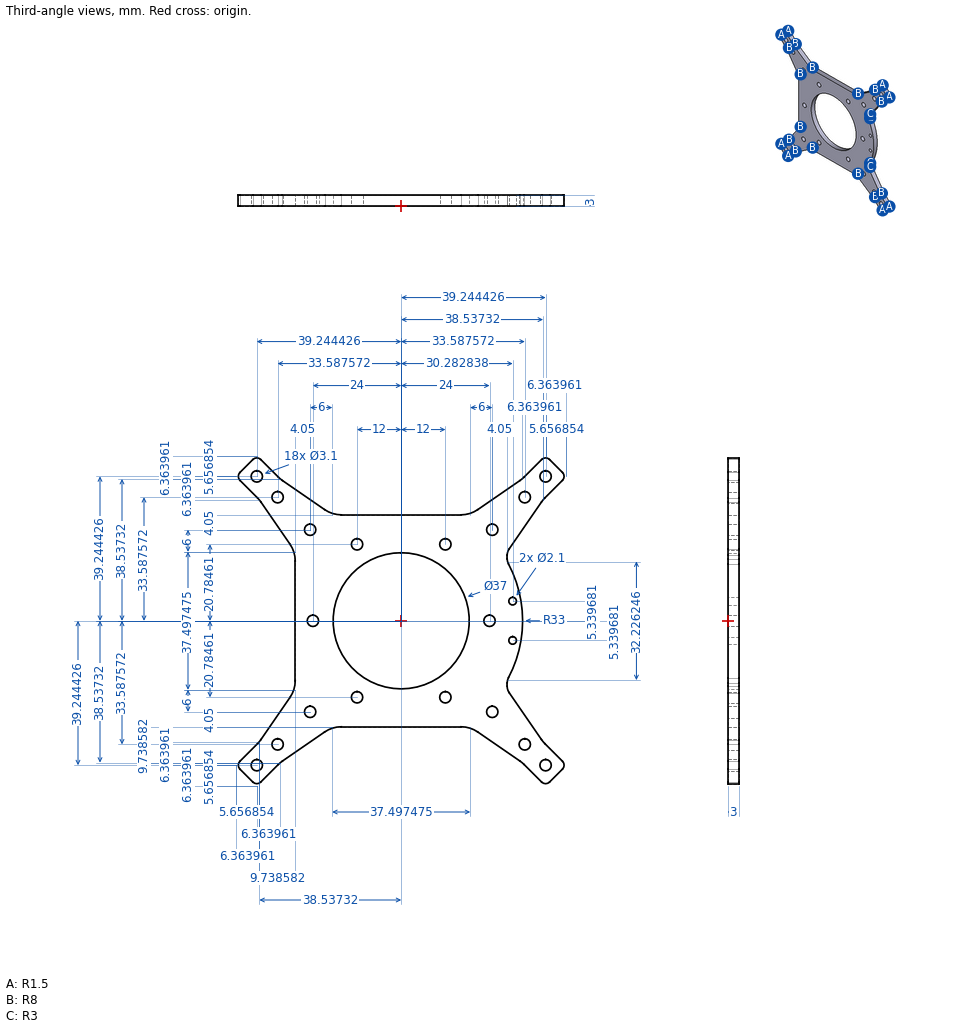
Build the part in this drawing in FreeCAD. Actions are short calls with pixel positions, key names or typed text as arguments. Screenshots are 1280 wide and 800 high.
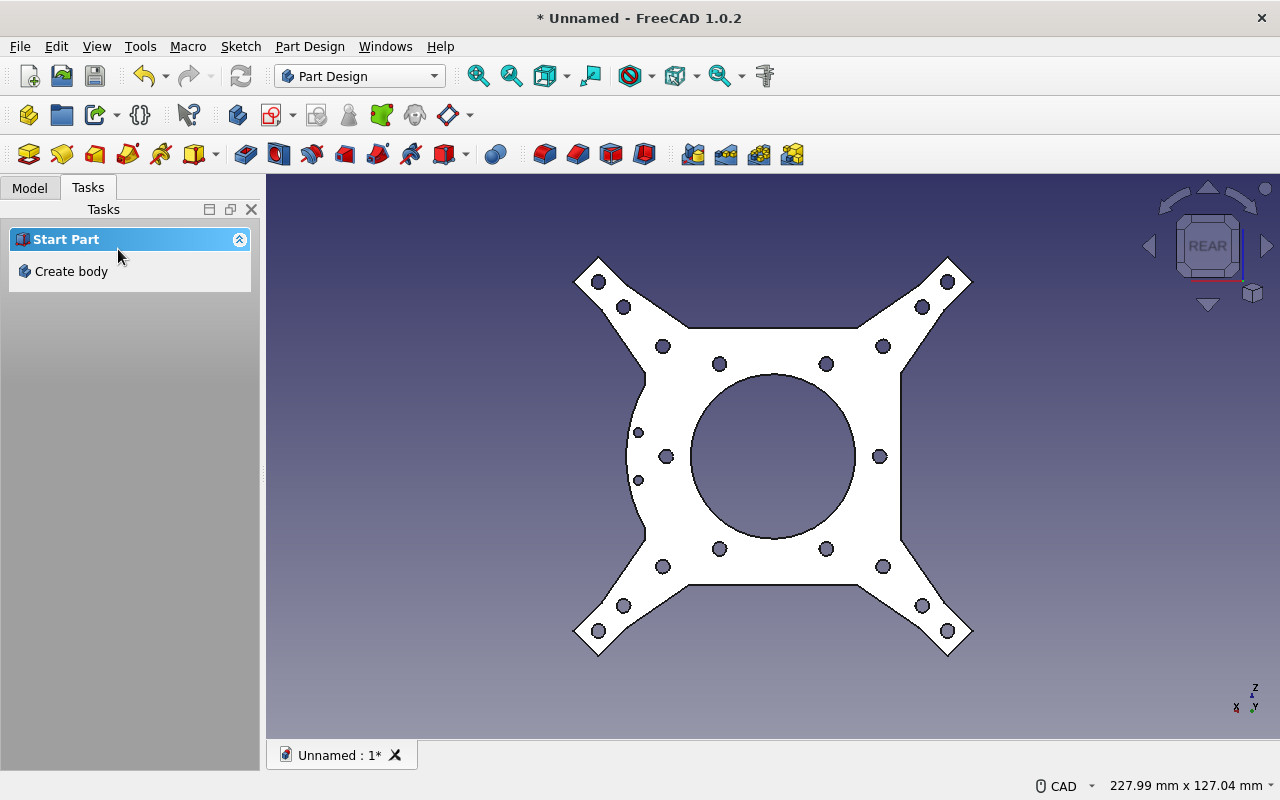
scroll(598, 655, up, 6)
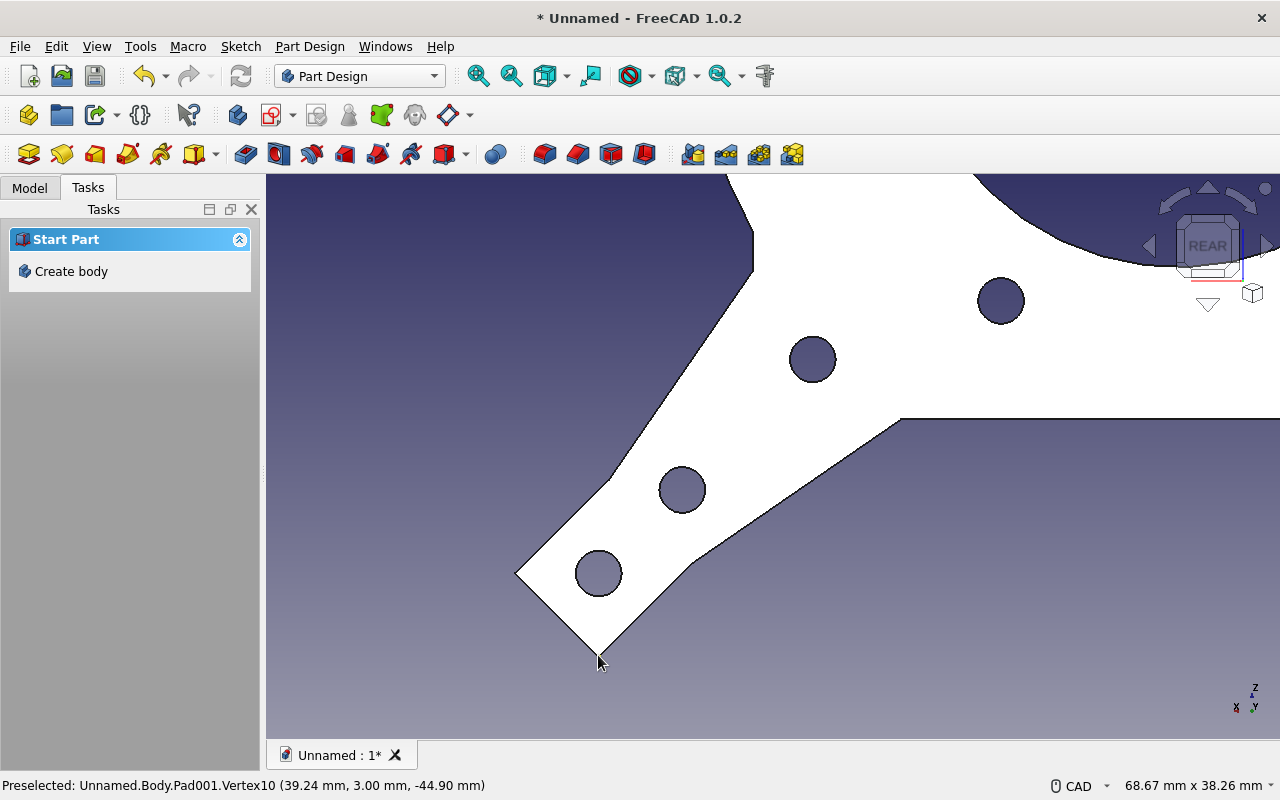
click(479, 76)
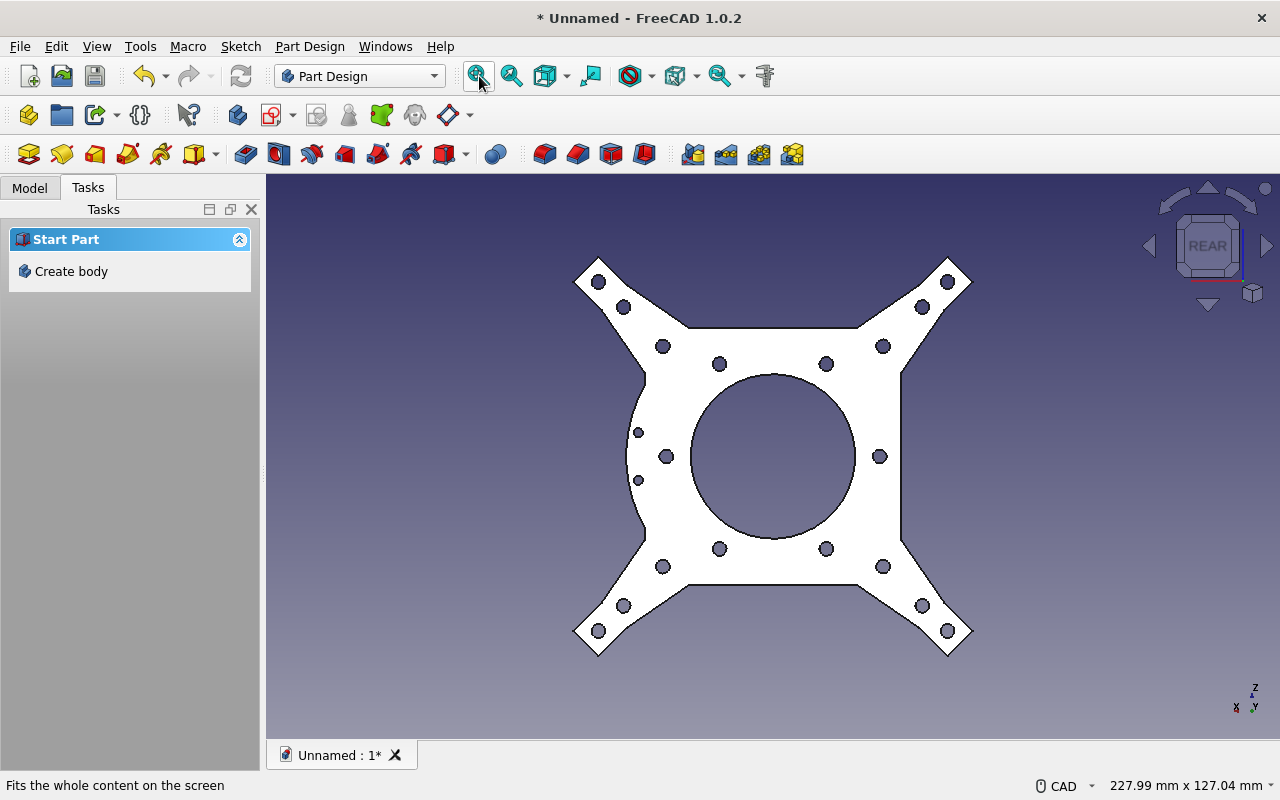
key(0)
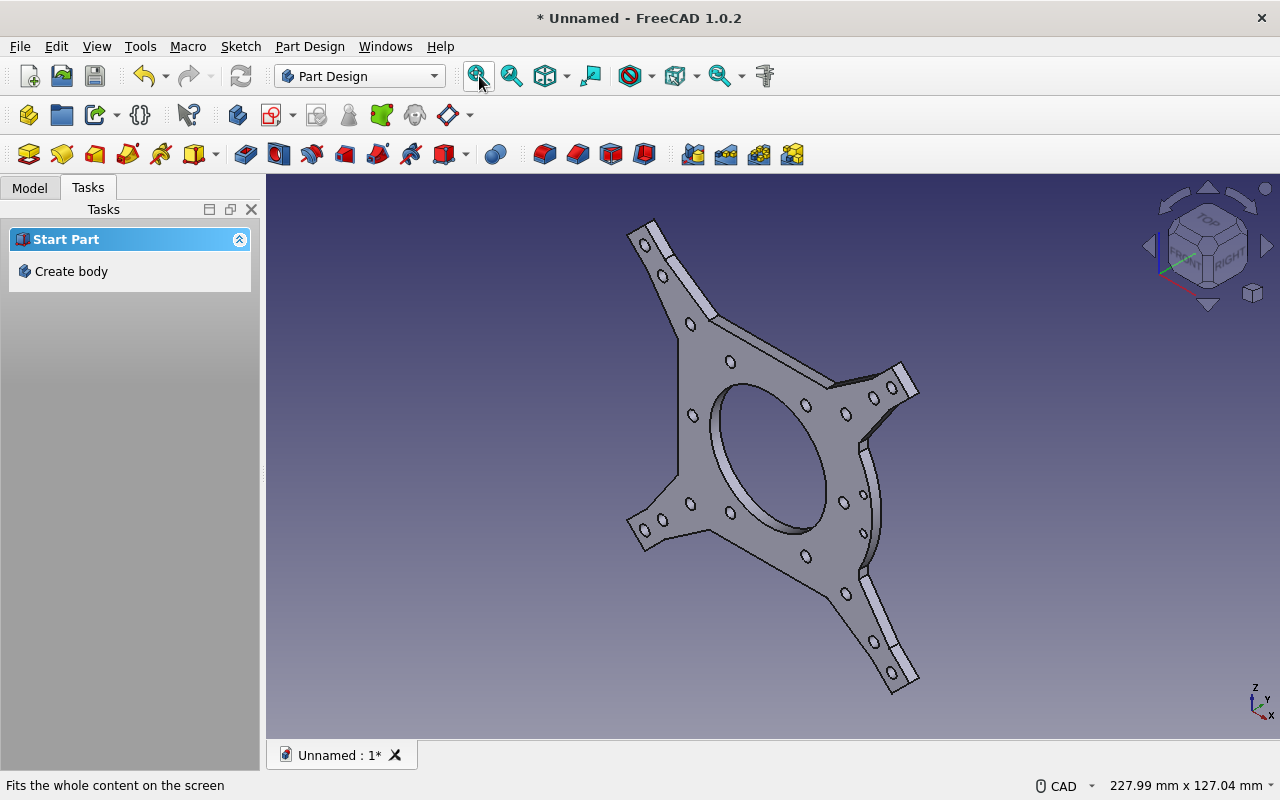
click(915, 679)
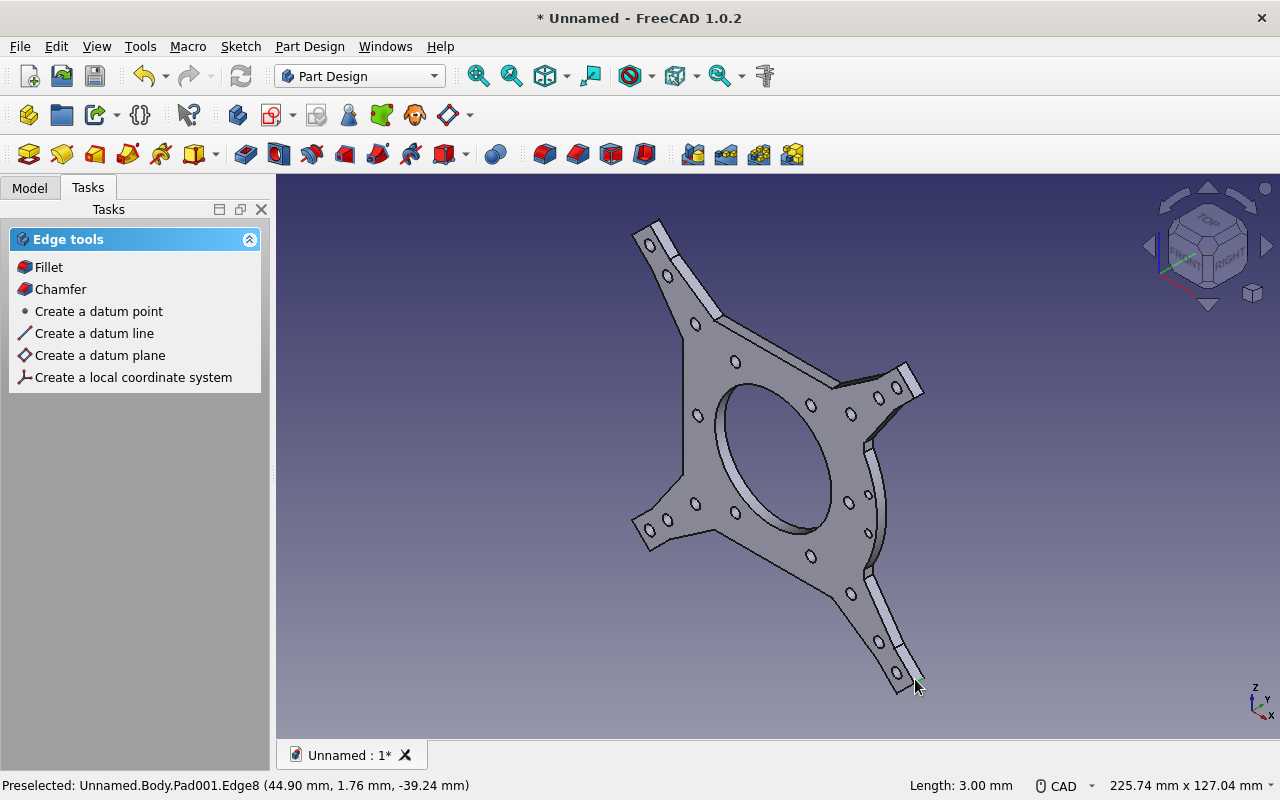
click(920, 394, ctrl)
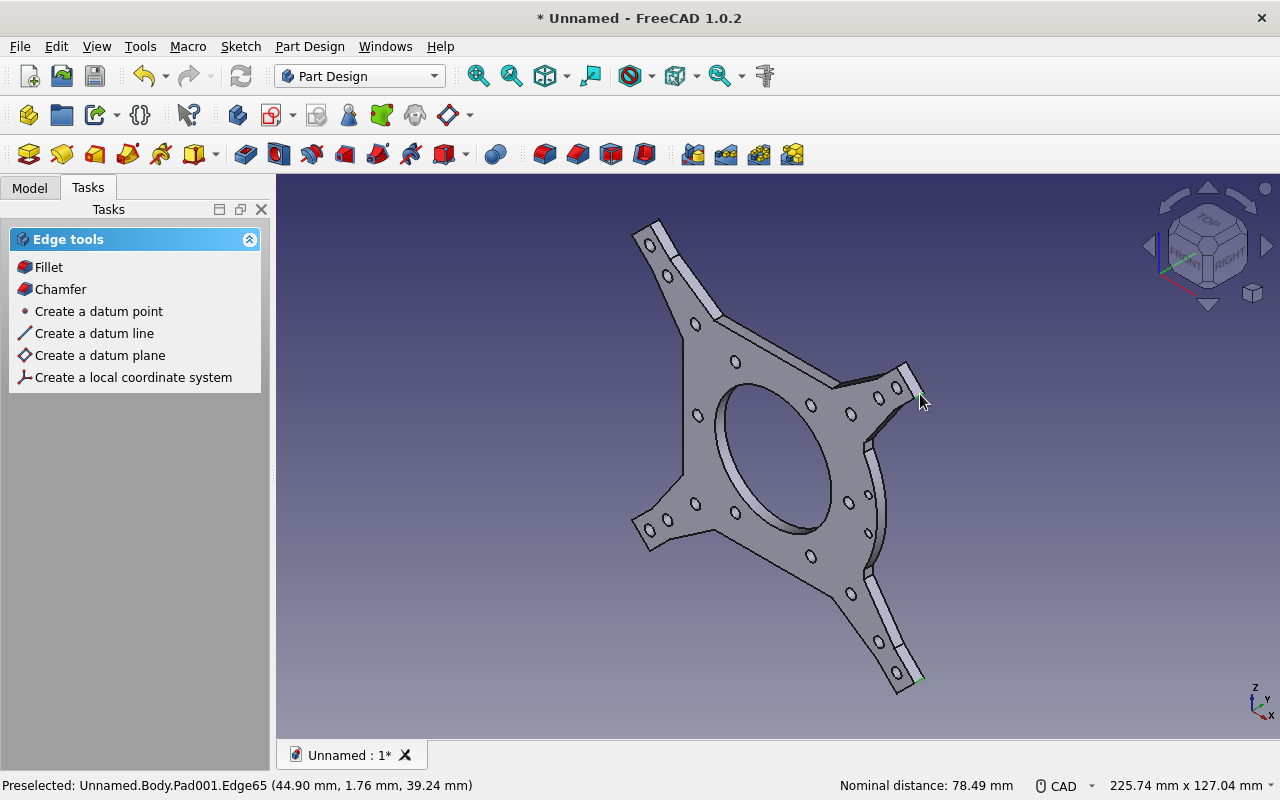
scroll(901, 690, up, 6)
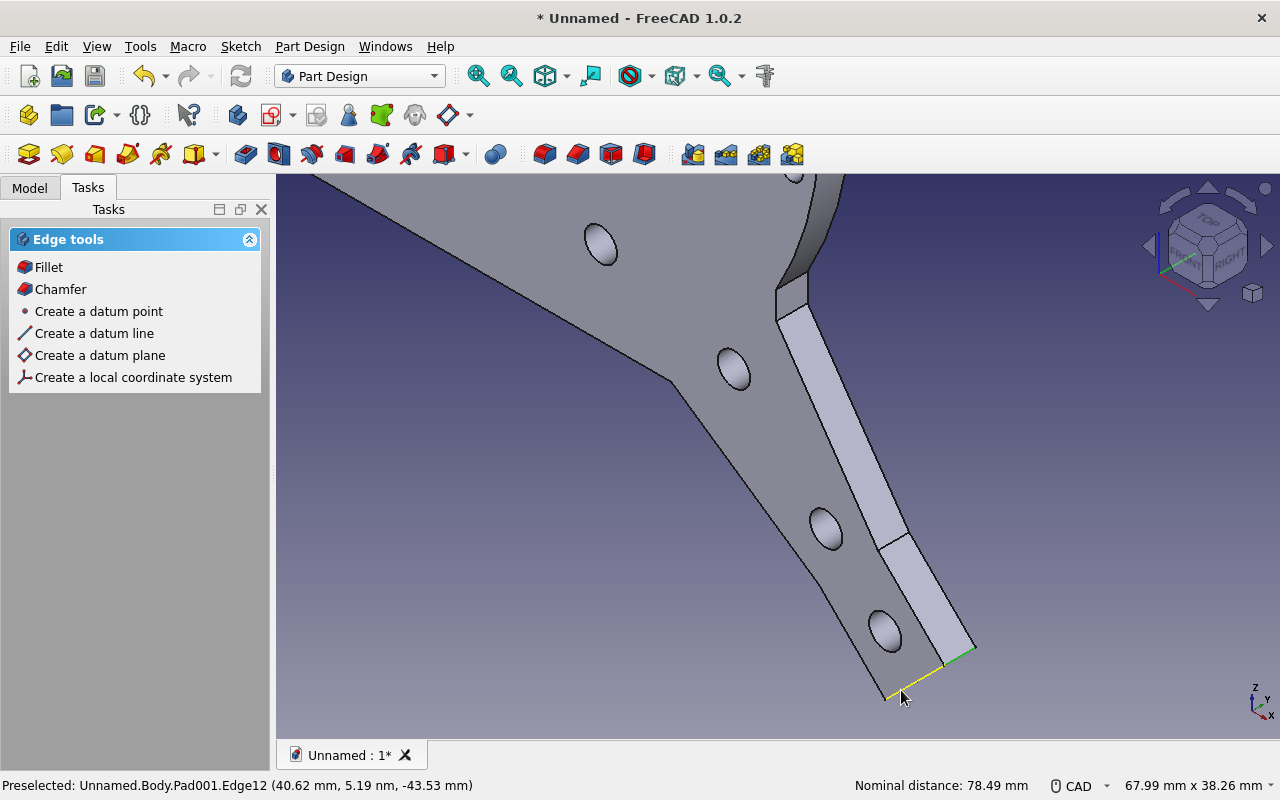
click(479, 76)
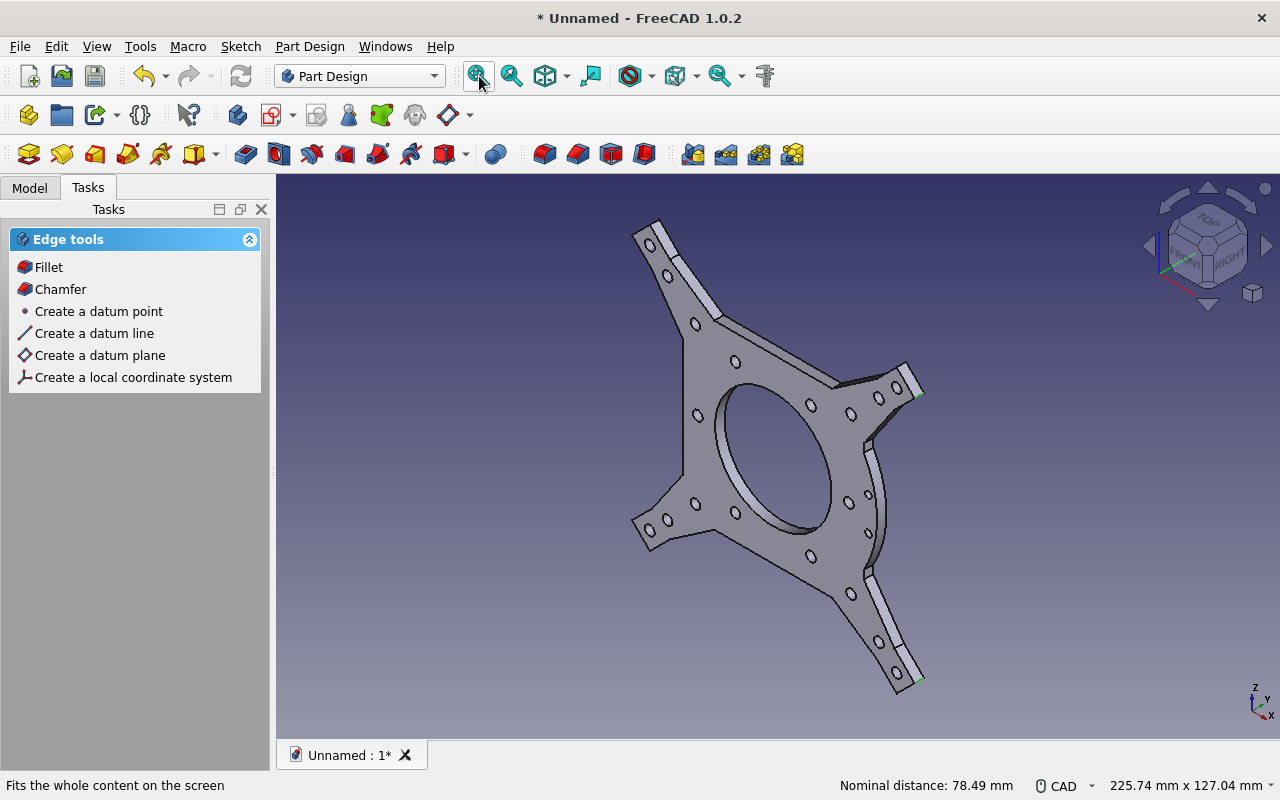
key(2)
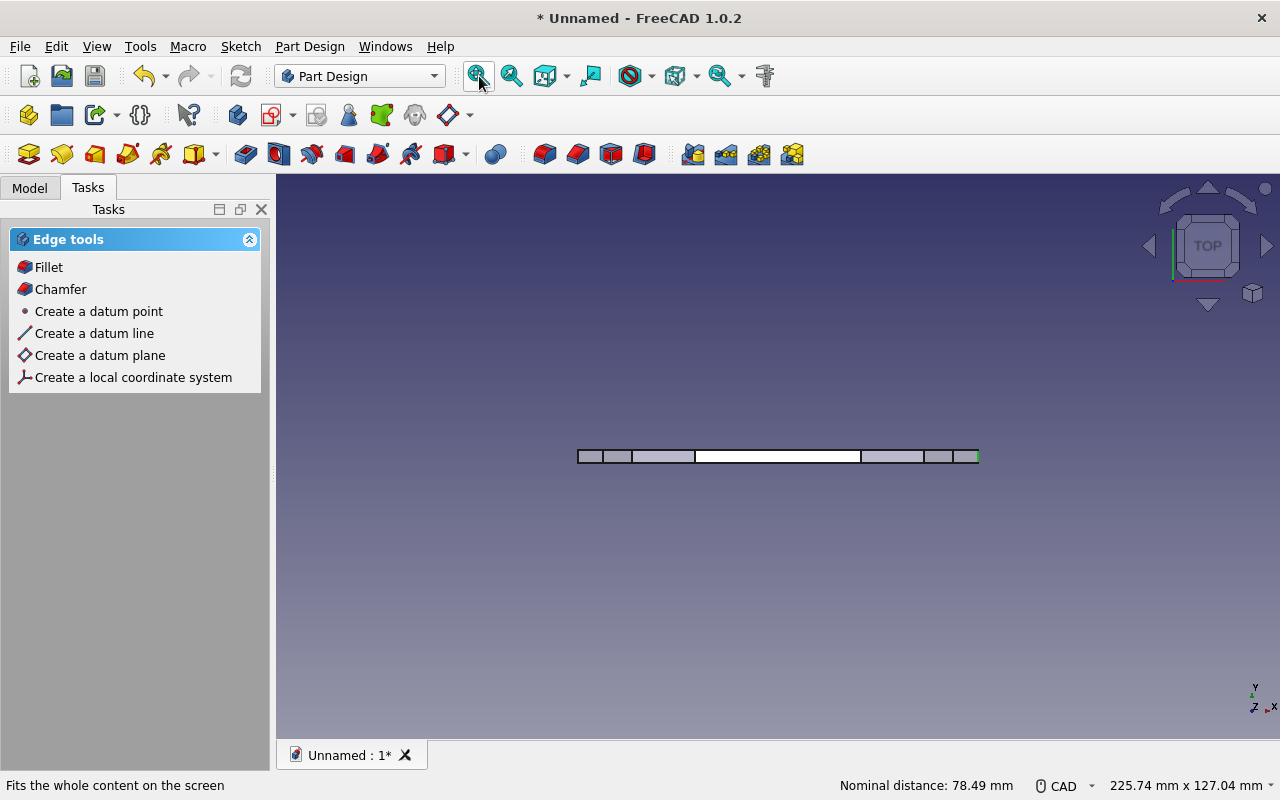
key(v)
key(f)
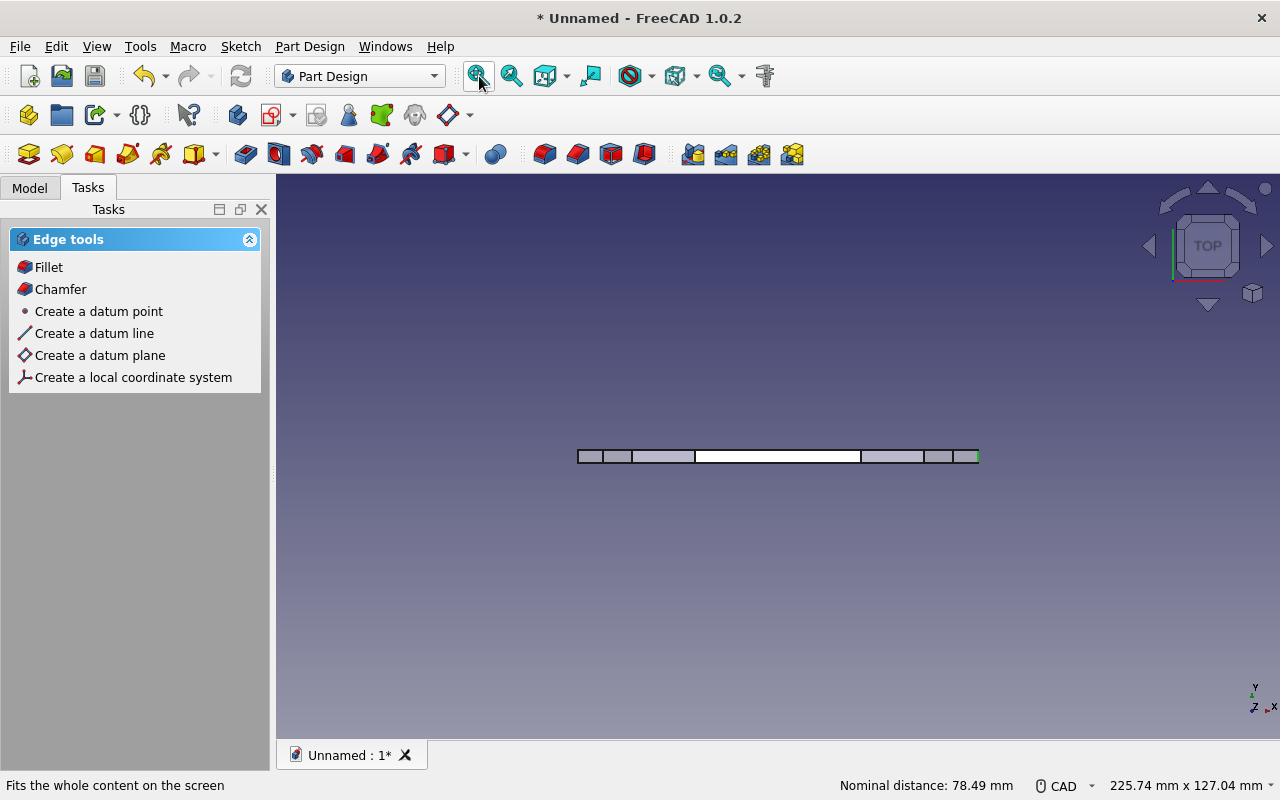
click(953, 455, ctrl)